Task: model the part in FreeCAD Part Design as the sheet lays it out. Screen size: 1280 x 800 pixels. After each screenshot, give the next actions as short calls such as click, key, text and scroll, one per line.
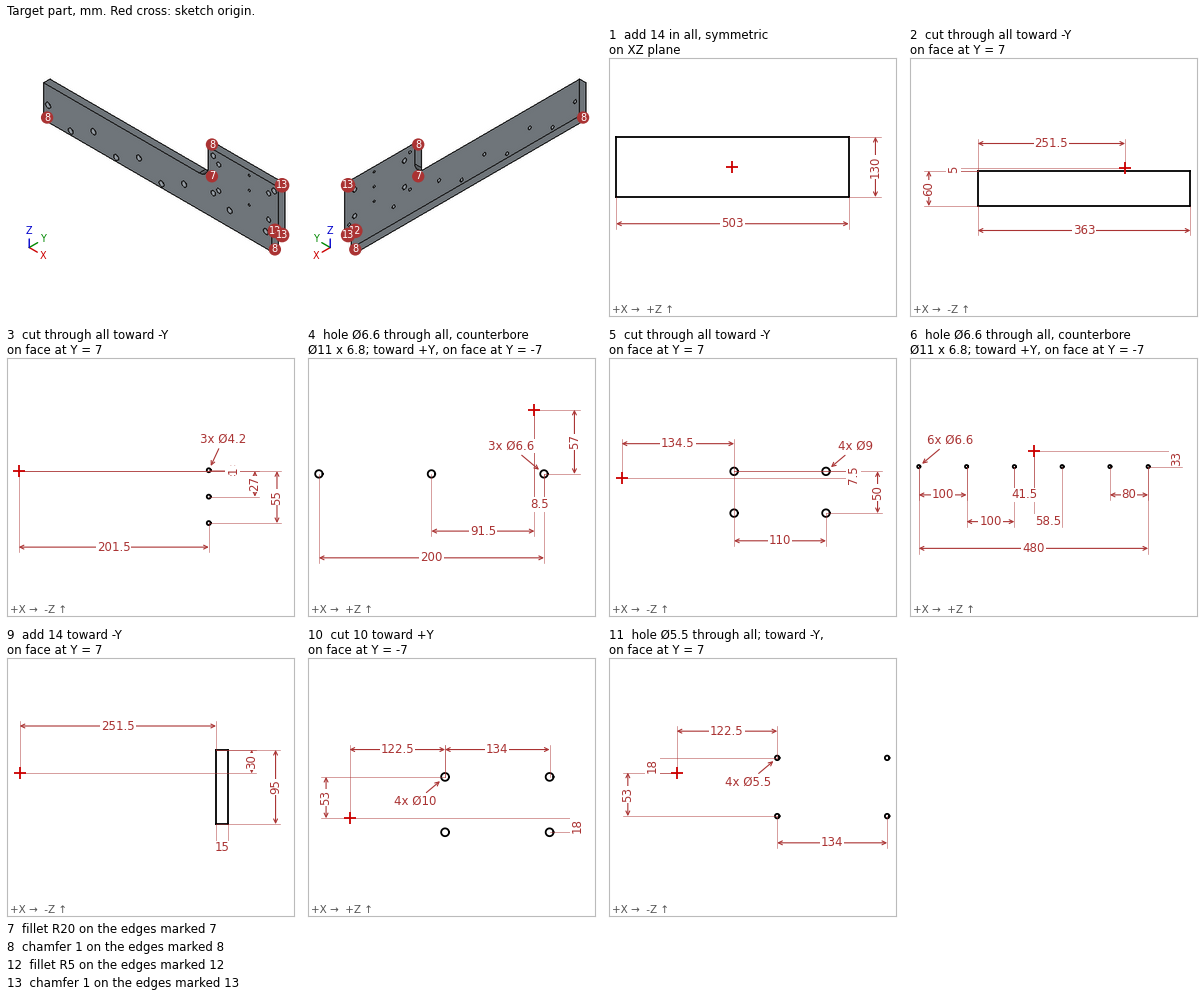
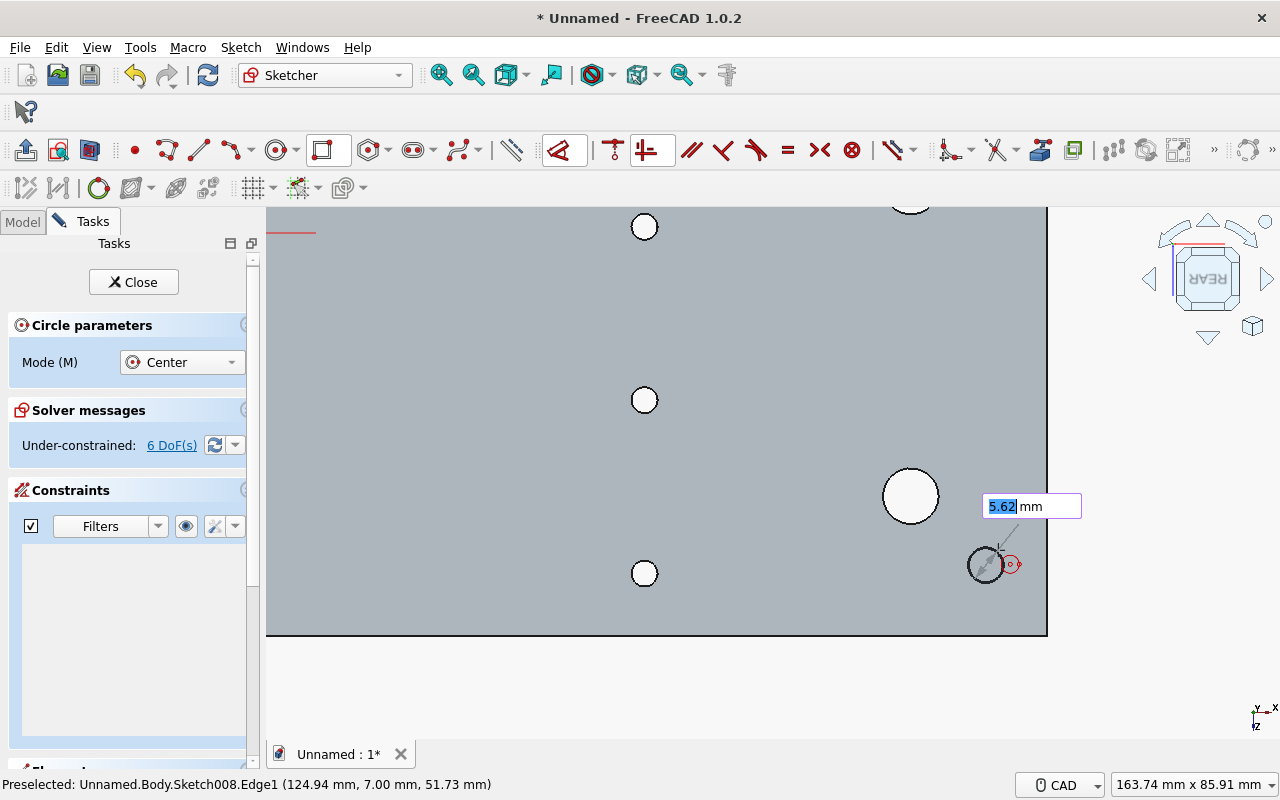
click(997, 549)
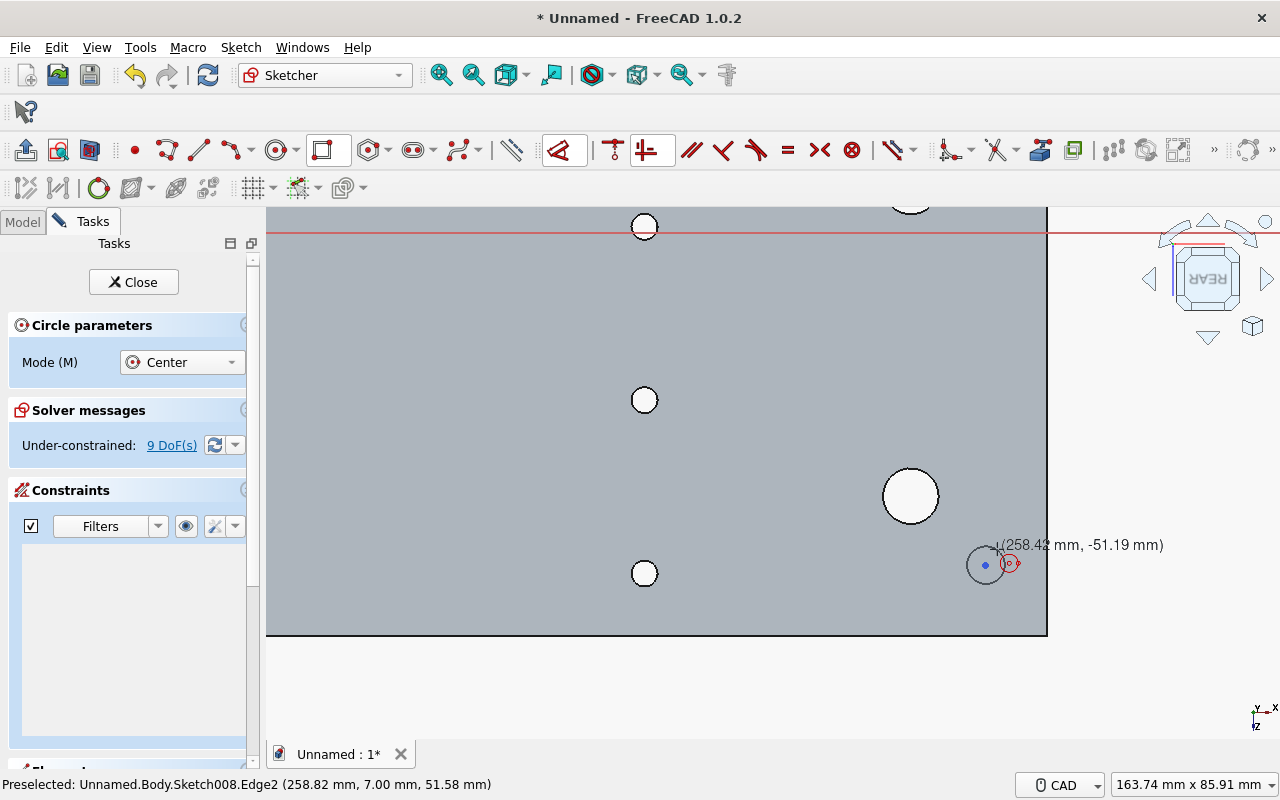
scroll(998, 550, down, 5)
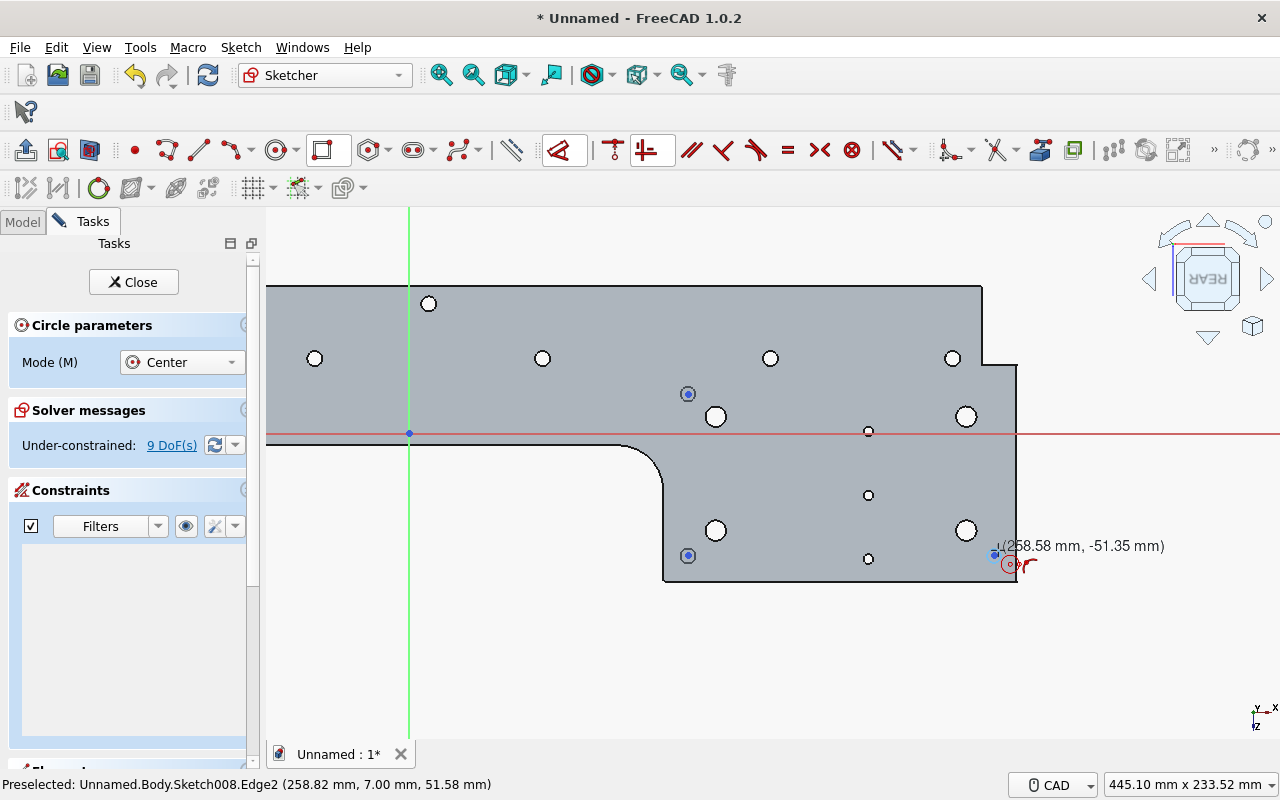
scroll(994, 393, up, 7)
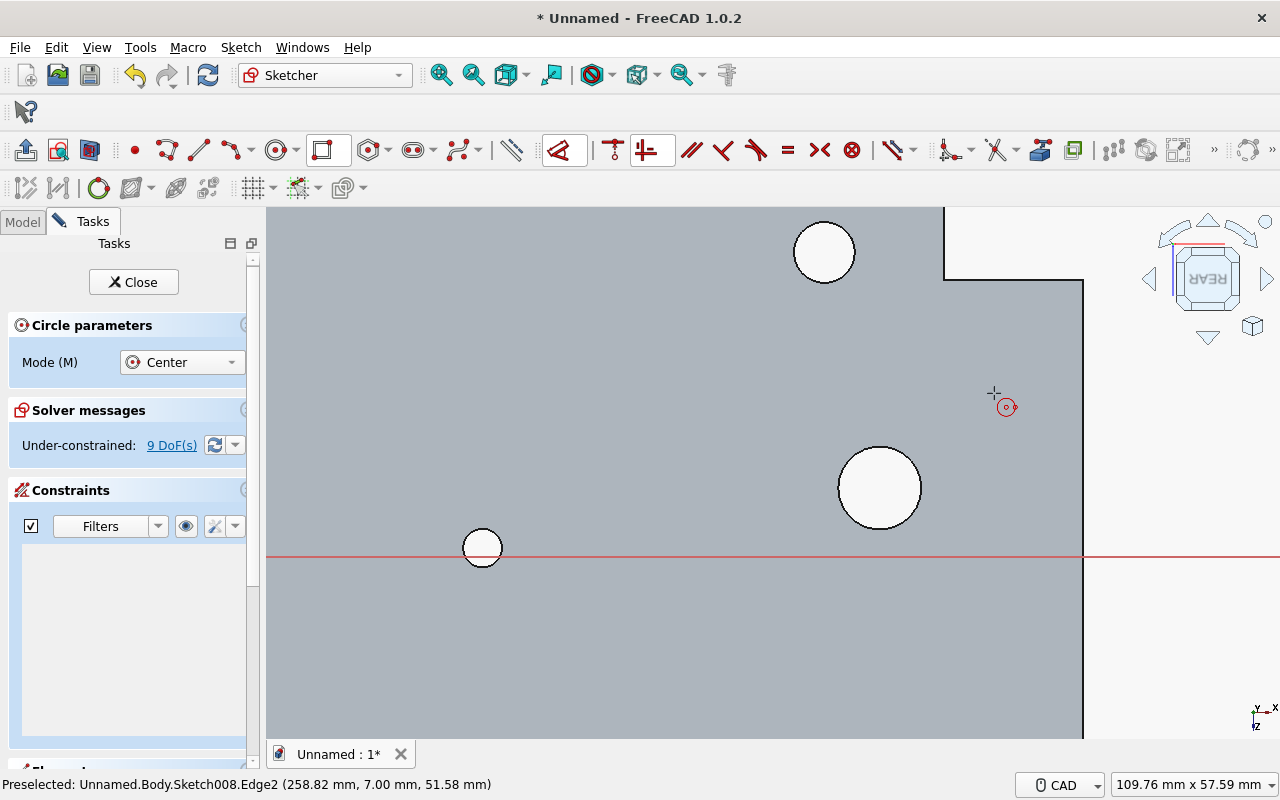
scroll(994, 392, down, 7)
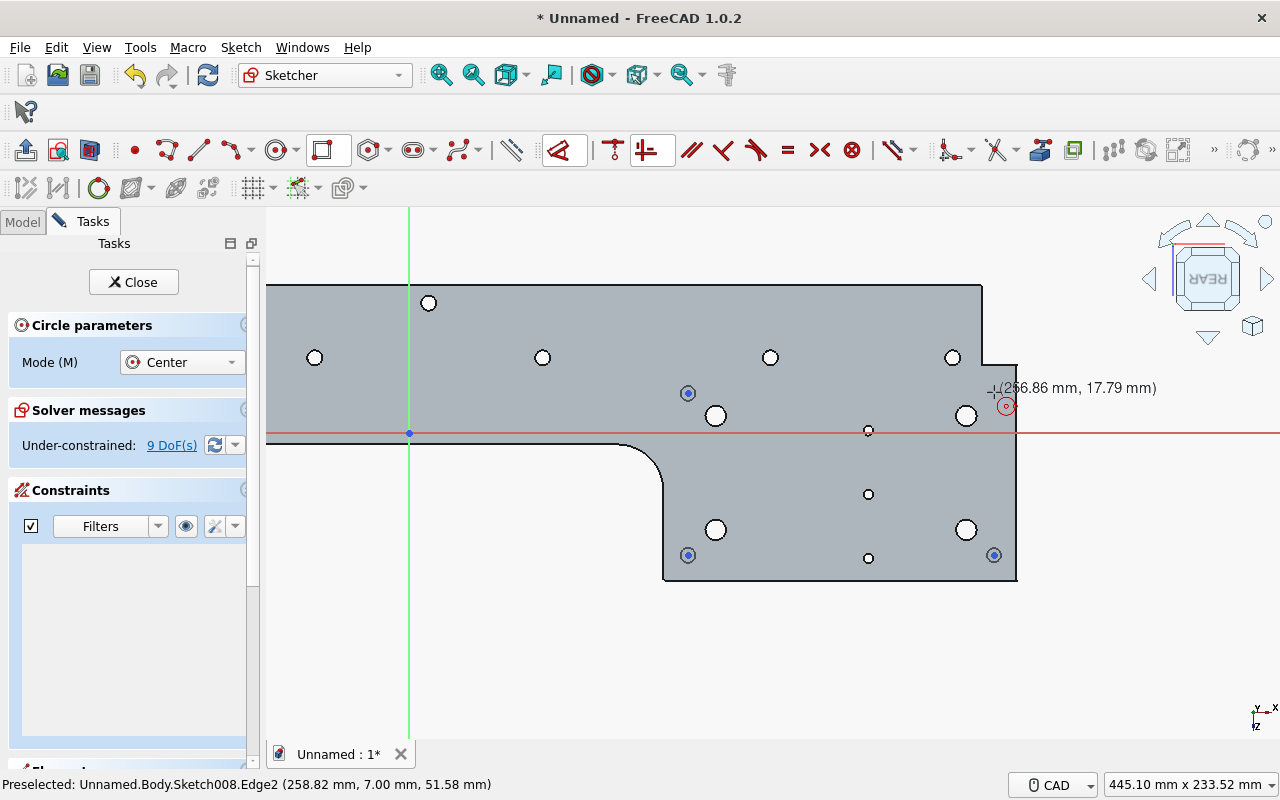
click(994, 392)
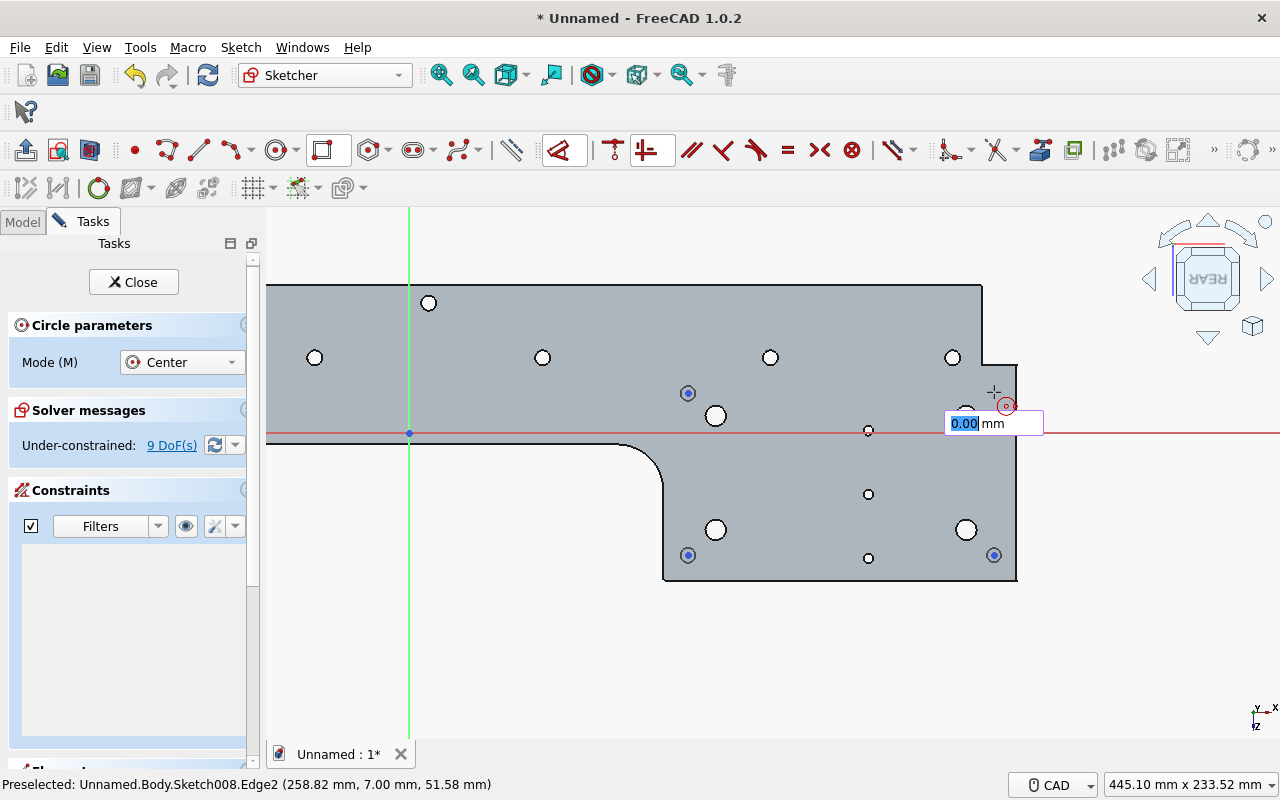
scroll(998, 388, up, 5)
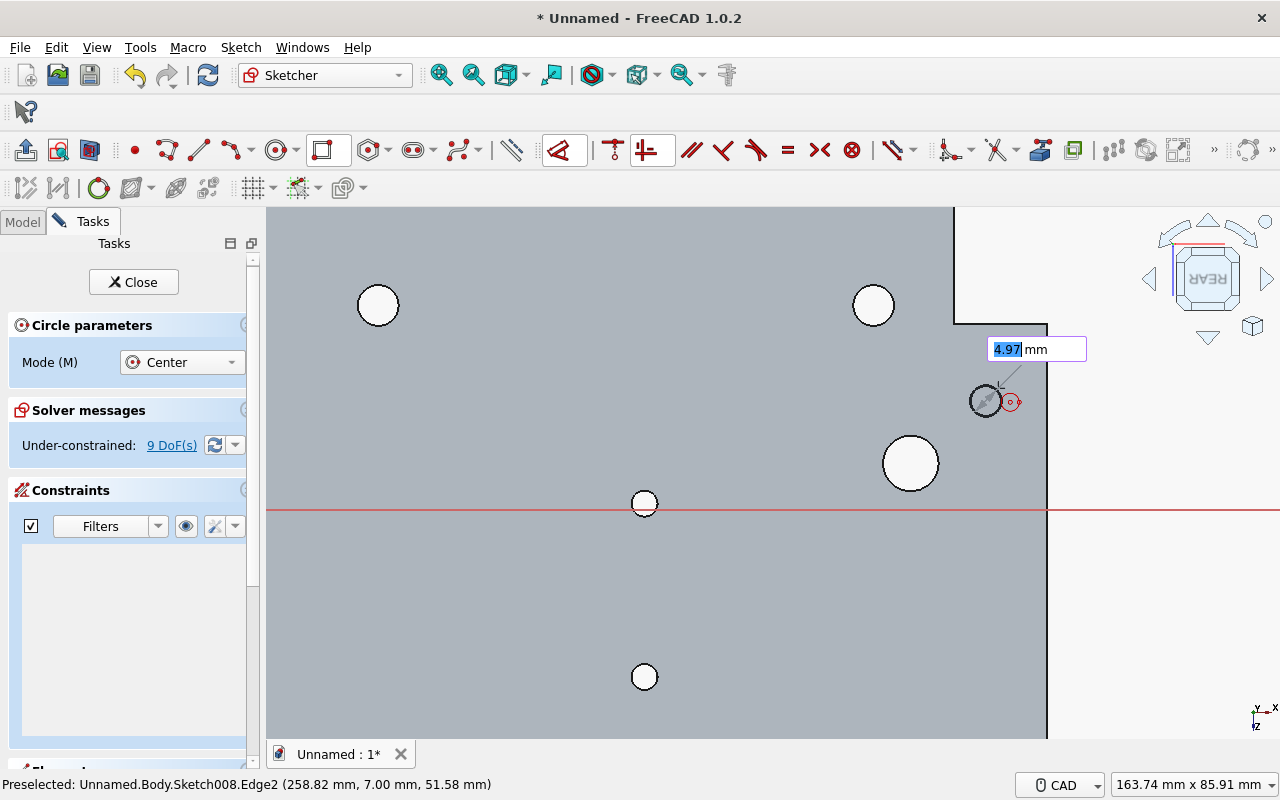
click(997, 386)
key(Escape)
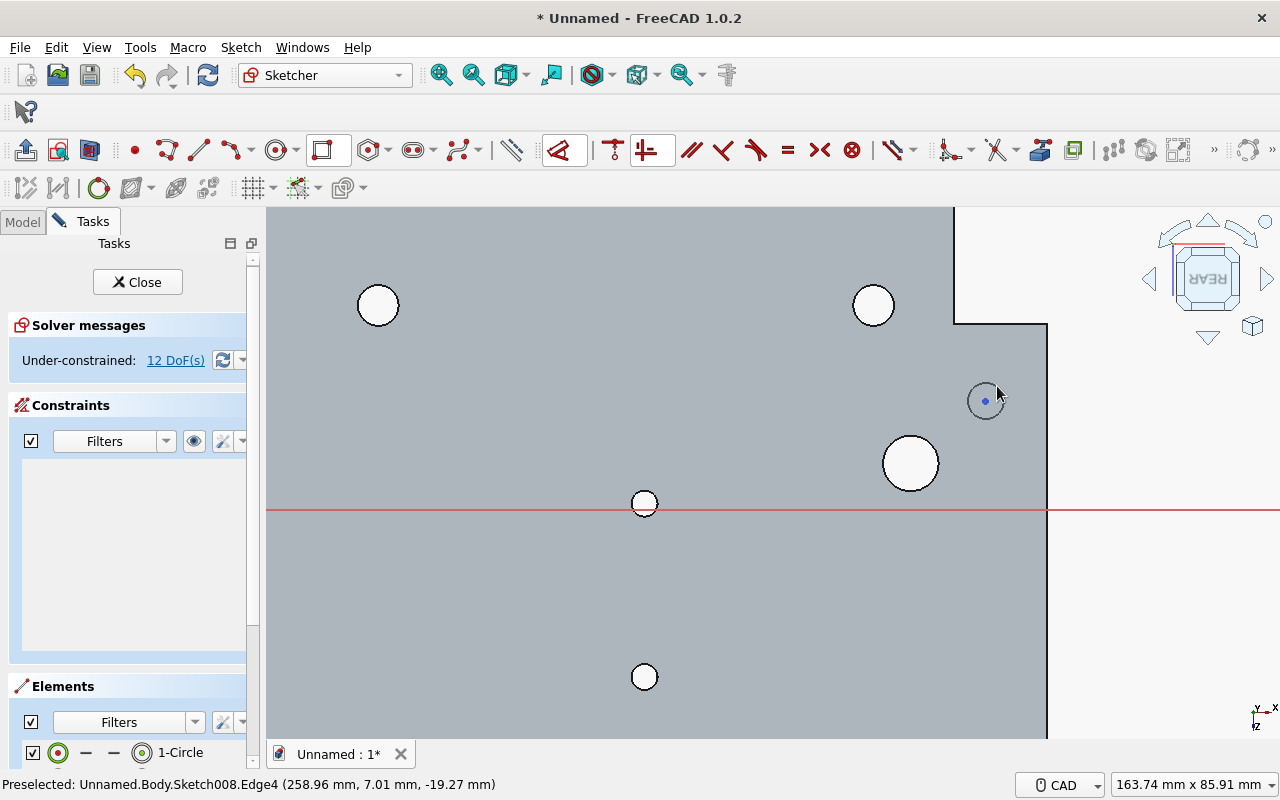
scroll(998, 389, down, 5)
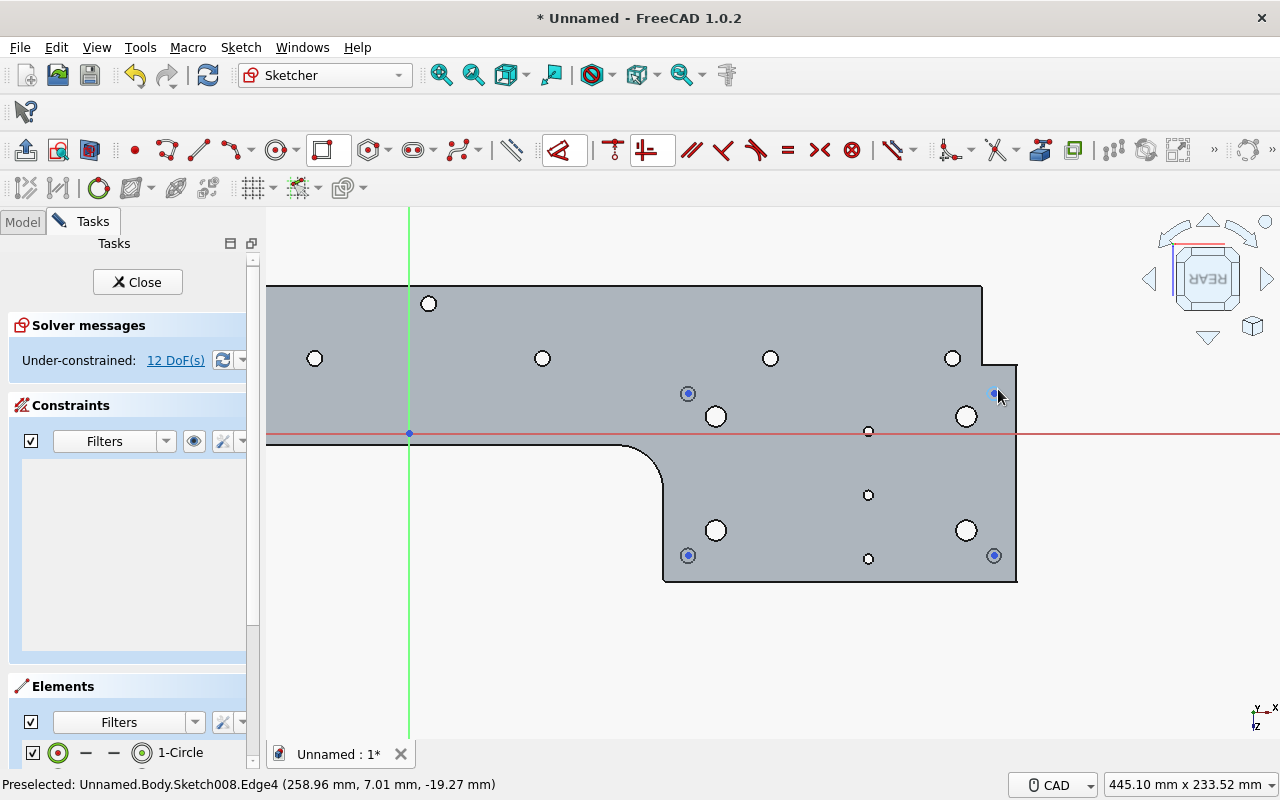
scroll(693, 389, up, 4)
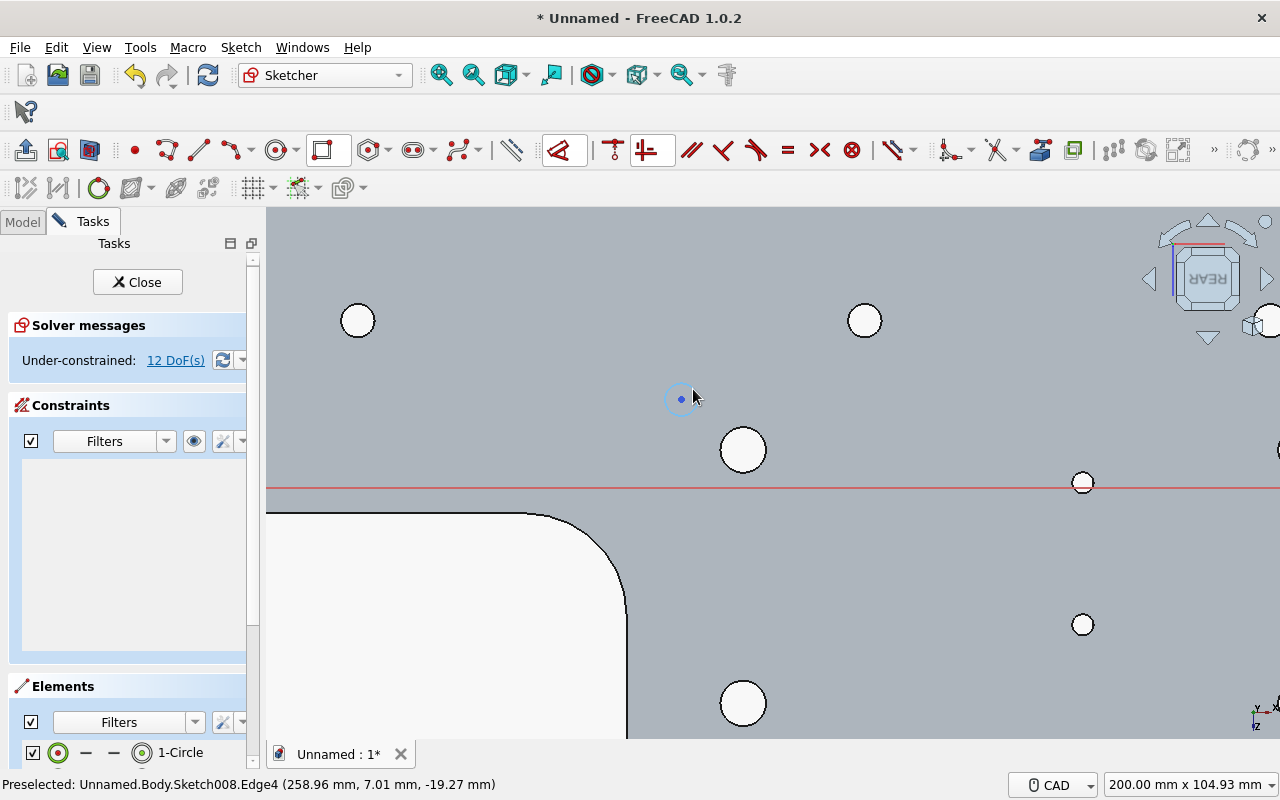
click(693, 388)